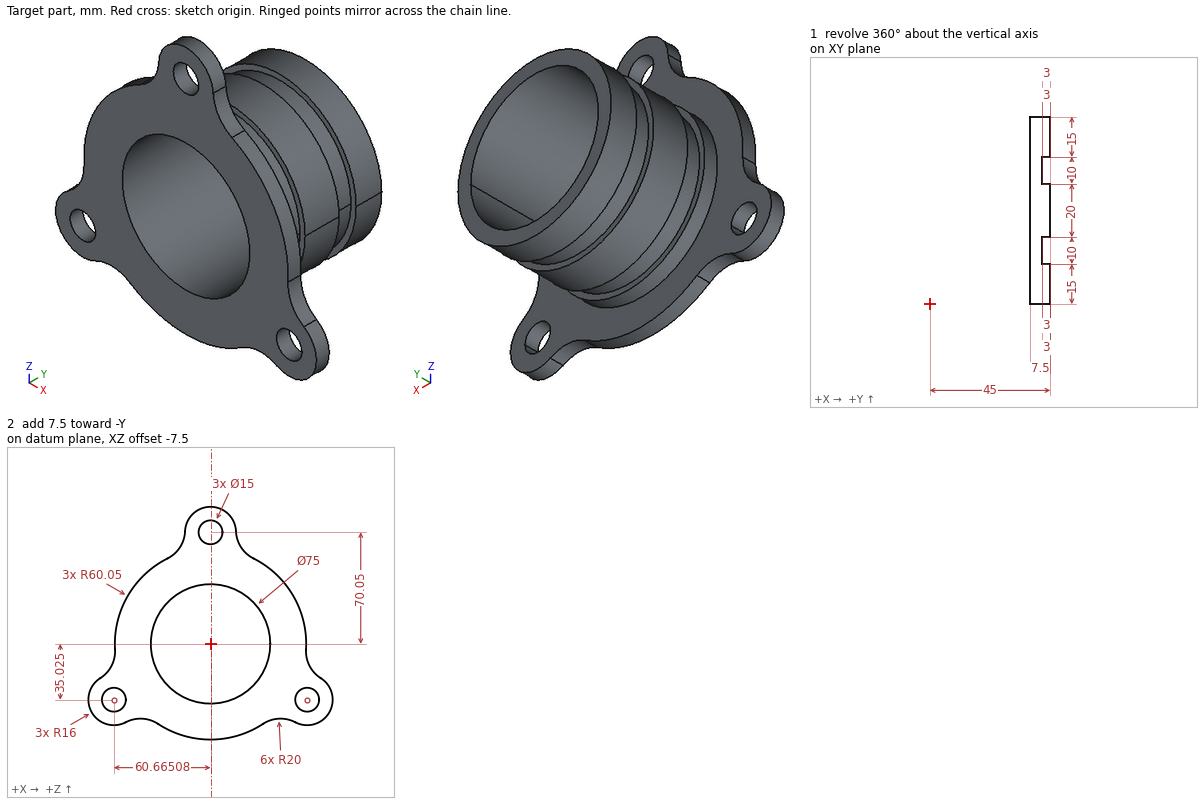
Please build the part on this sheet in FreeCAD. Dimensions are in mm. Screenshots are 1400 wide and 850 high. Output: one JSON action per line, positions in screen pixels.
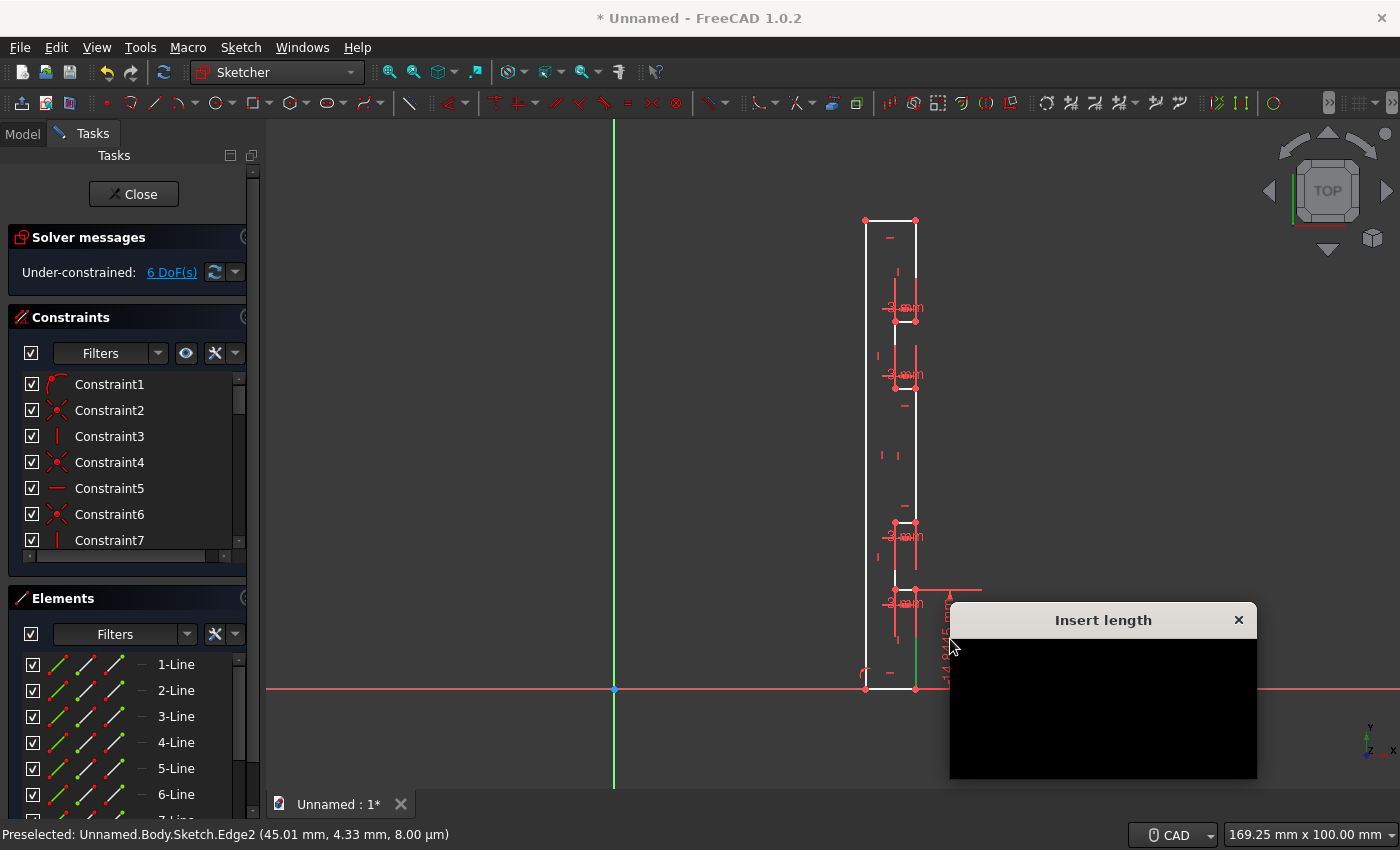
{"action": "type", "text": "15"}
{"action": "key", "text": "Return"}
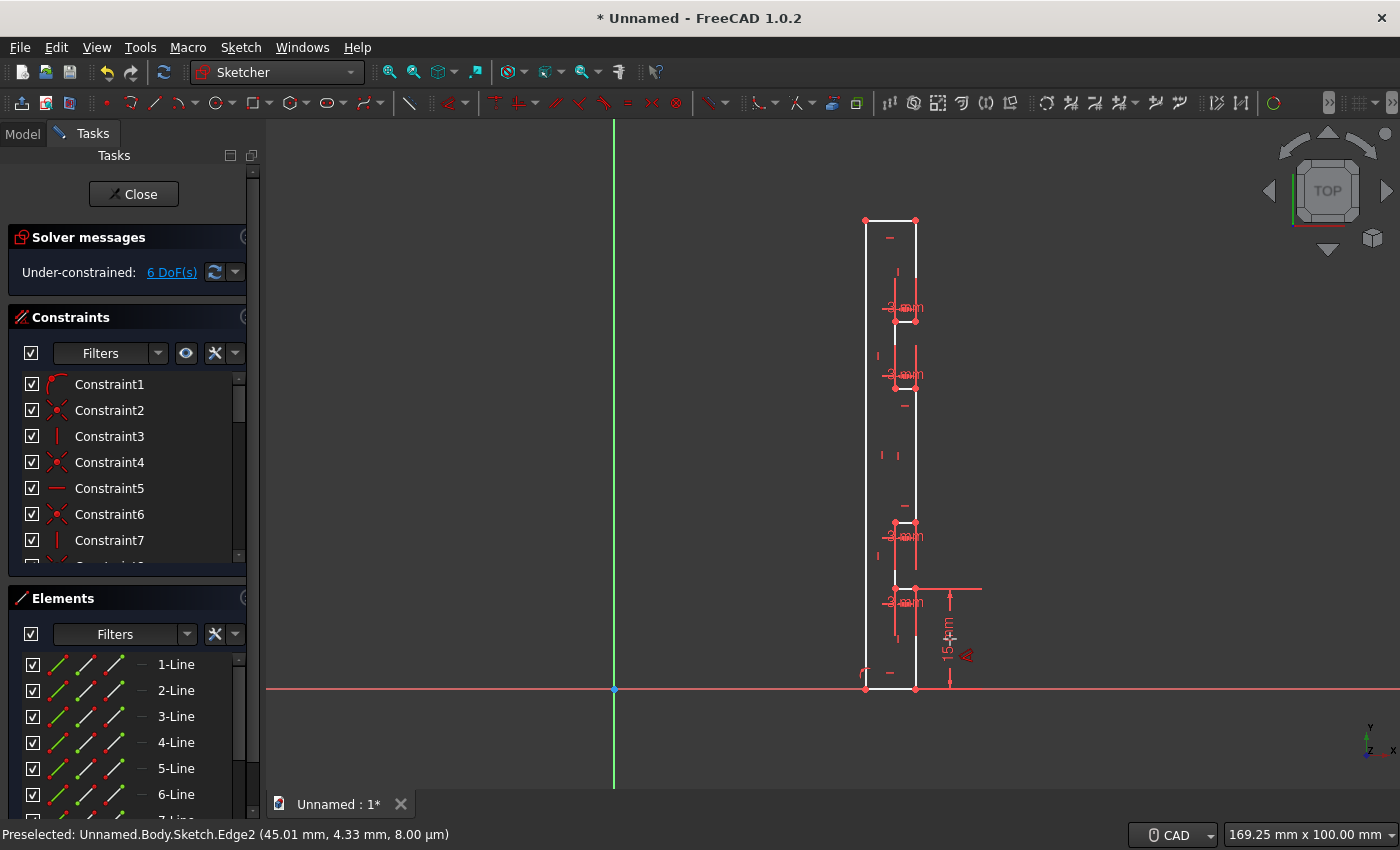
{"action": "left_click", "coordinate": [895, 569]}
{"action": "left_click", "coordinate": [929, 571]}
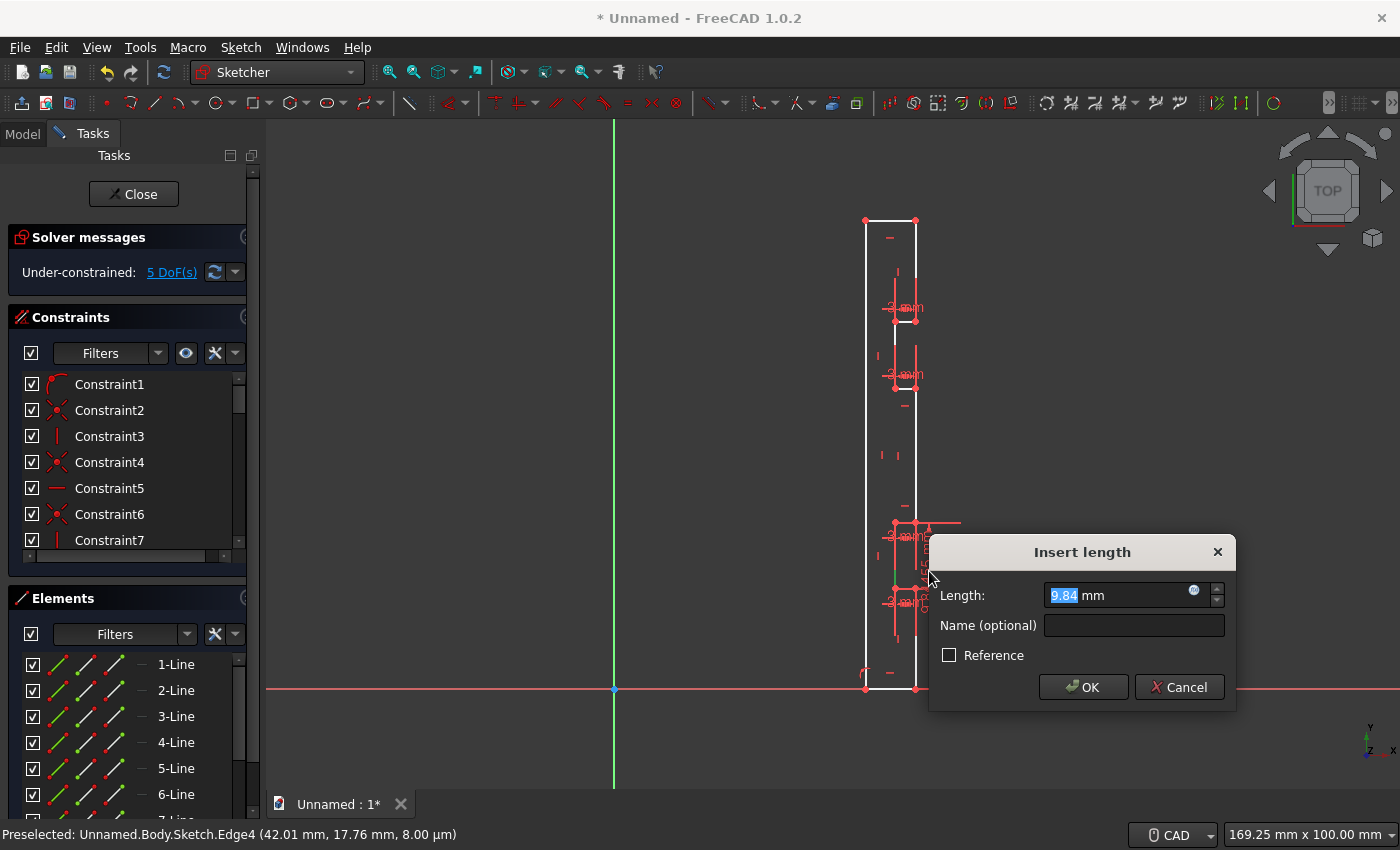
{"action": "type", "text": "10"}
{"action": "key", "text": "Return"}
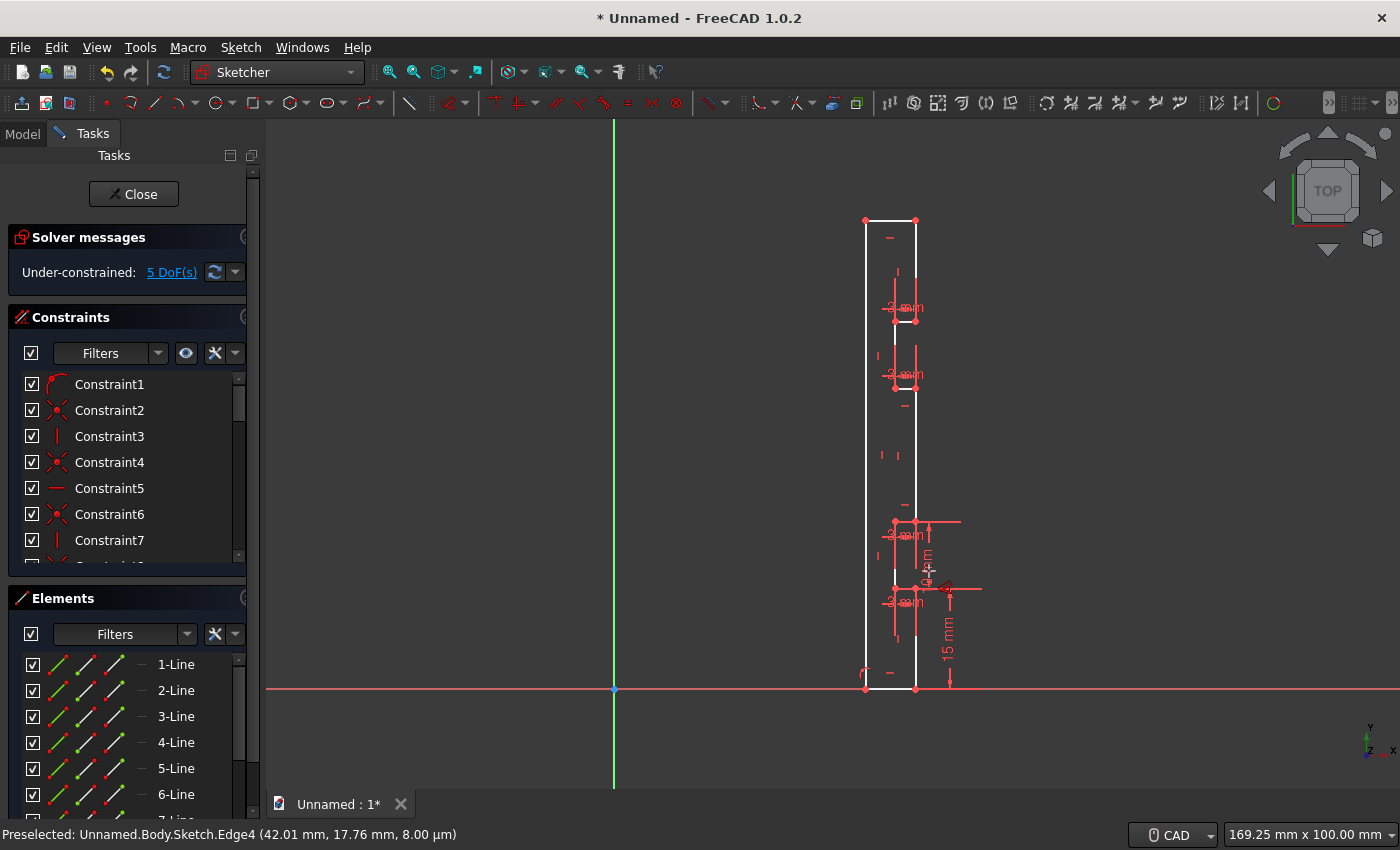
{"action": "left_click", "coordinate": [916, 482]}
{"action": "left_click", "coordinate": [950, 455]}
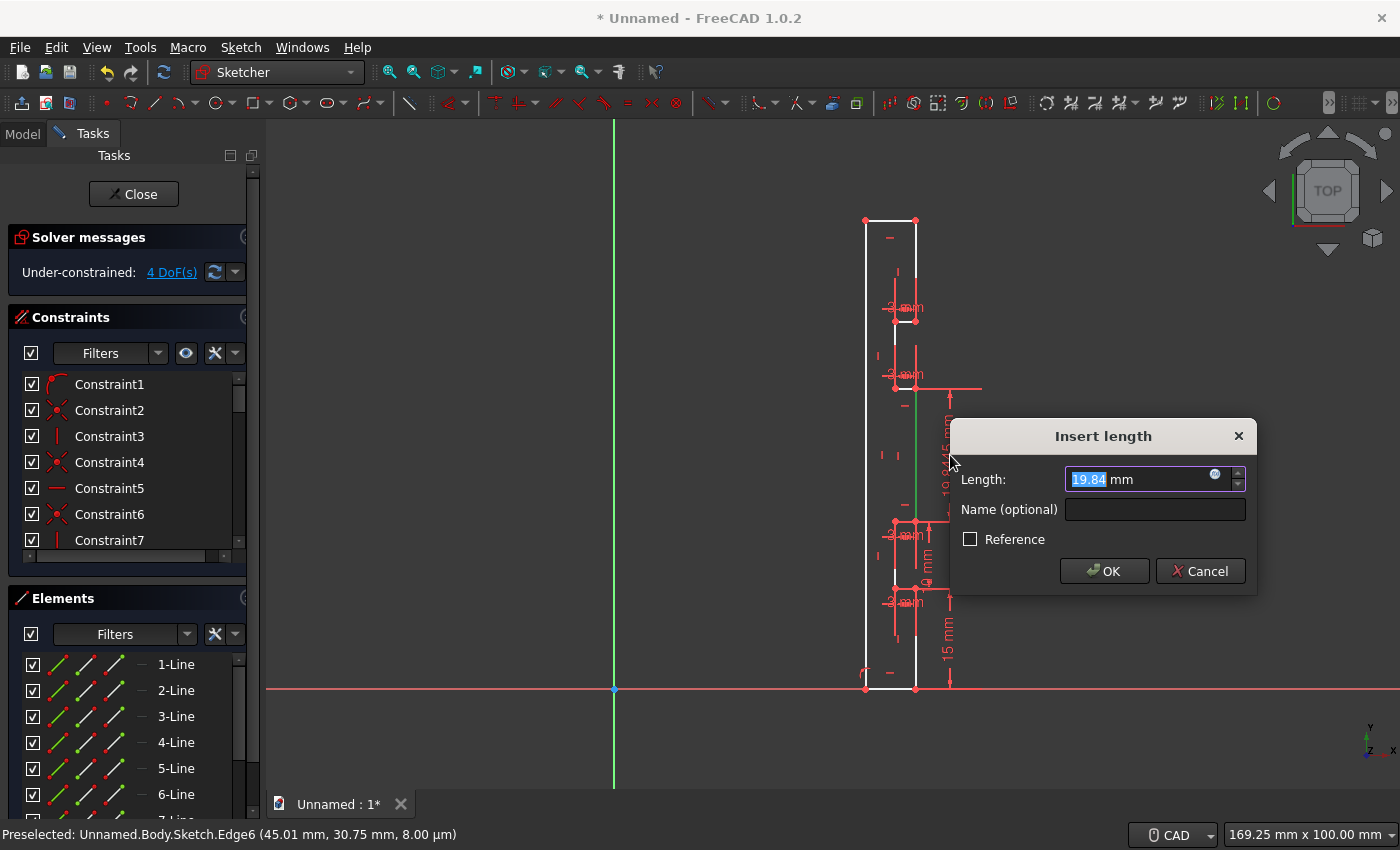
{"action": "type", "text": "20"}
{"action": "key", "text": "Return"}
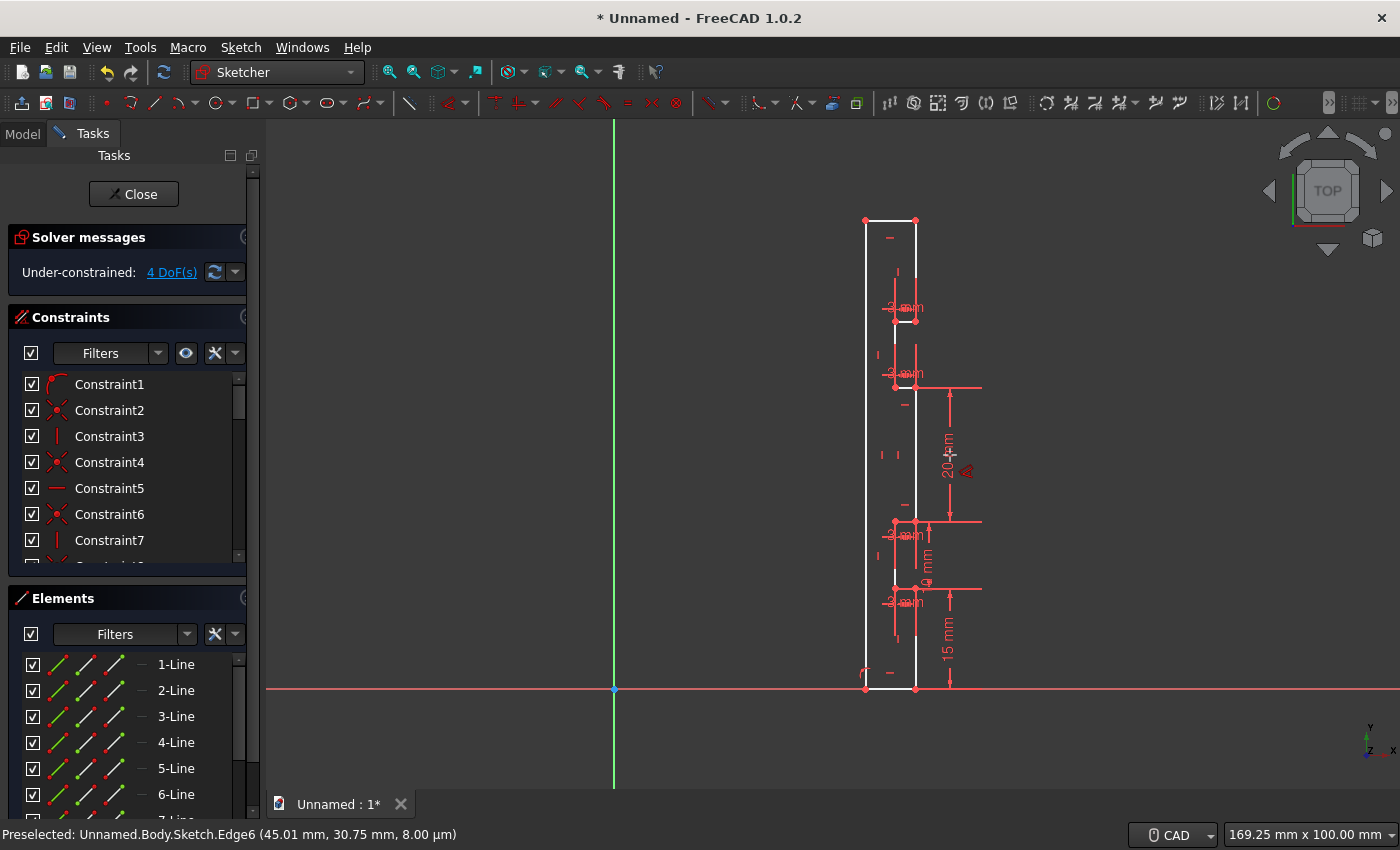
{"action": "left_click", "coordinate": [895, 368]}
{"action": "left_click", "coordinate": [929, 355]}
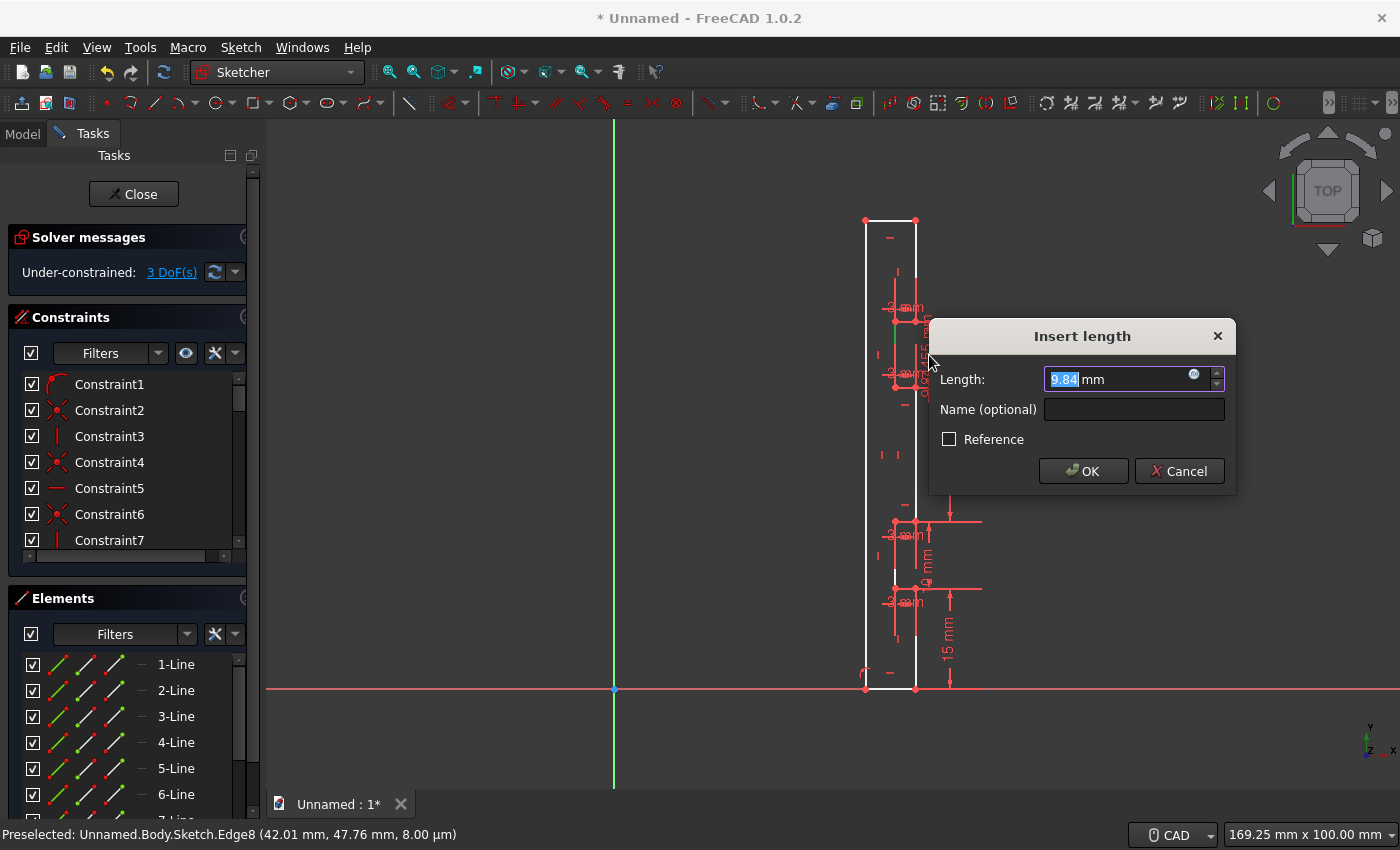
{"action": "type", "text": "10"}
{"action": "key", "text": "Return"}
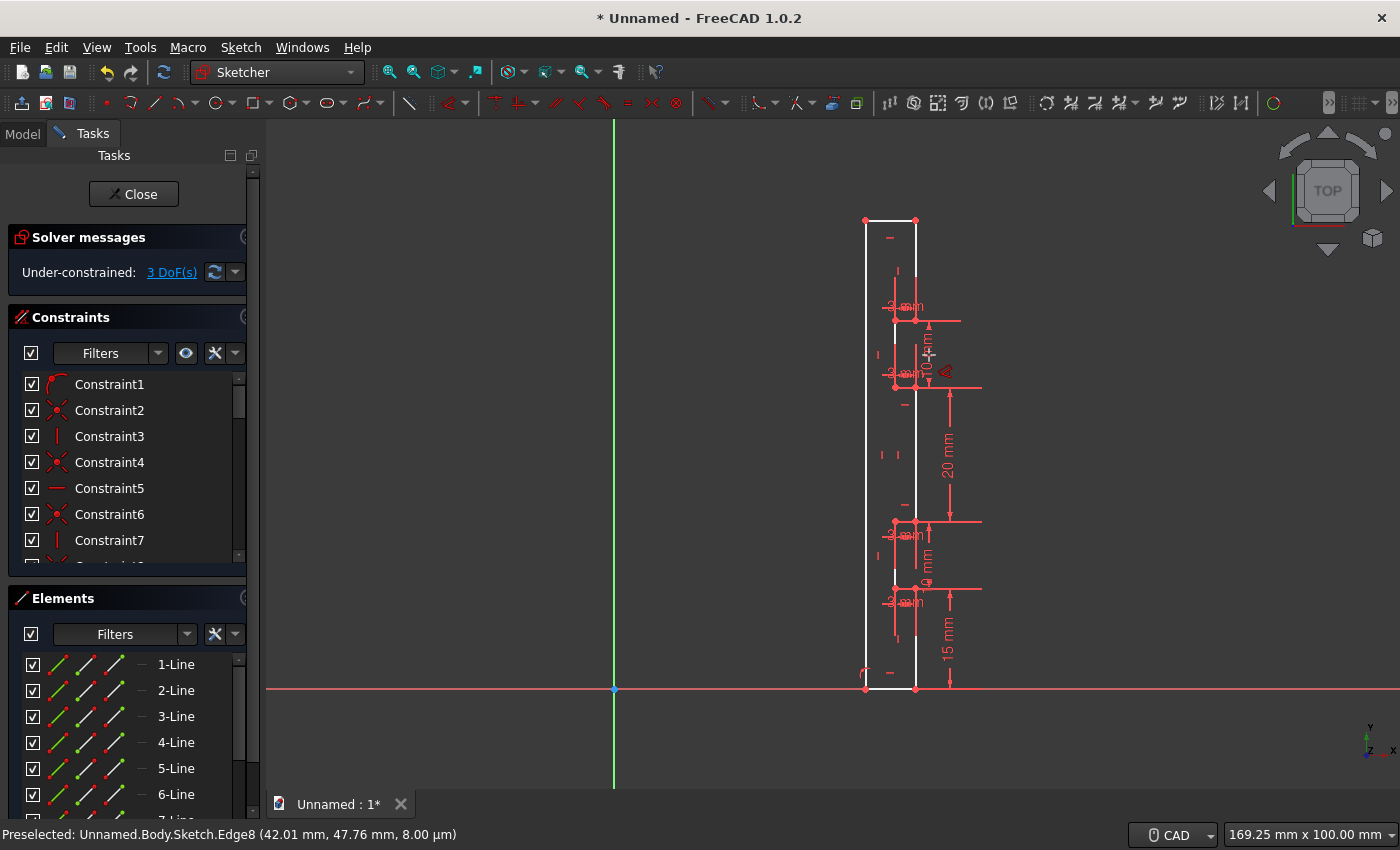
{"action": "left_click", "coordinate": [916, 291]}
{"action": "left_click", "coordinate": [950, 271]}